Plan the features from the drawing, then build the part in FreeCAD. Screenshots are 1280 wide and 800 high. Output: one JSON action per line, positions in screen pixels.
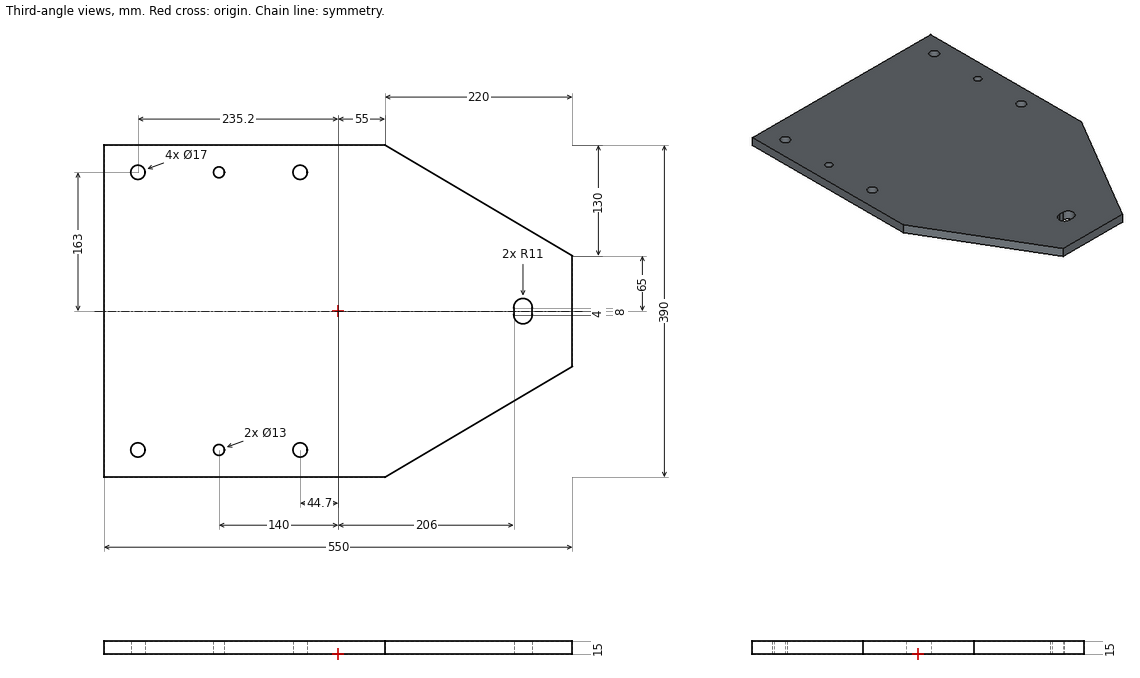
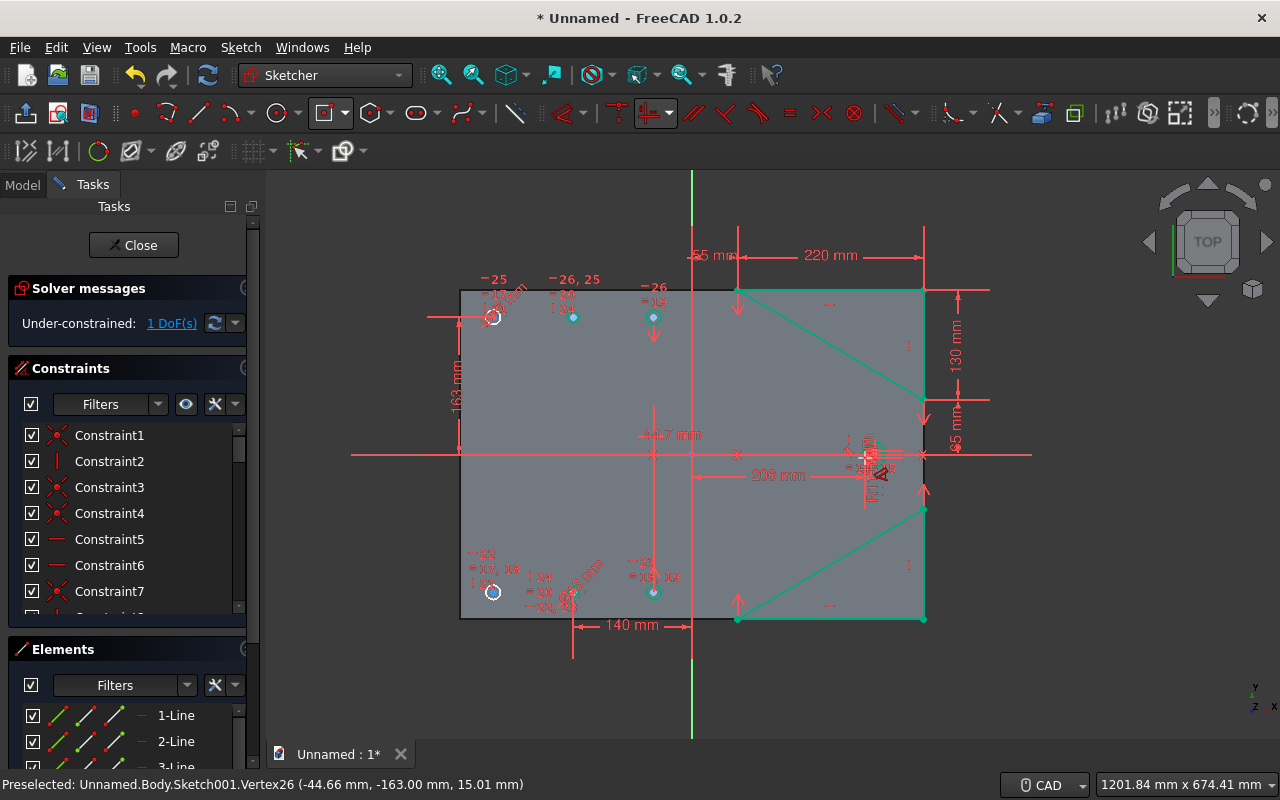
{"action": "left_click", "coordinate": [493, 317]}
{"action": "left_click", "coordinate": [592, 283]}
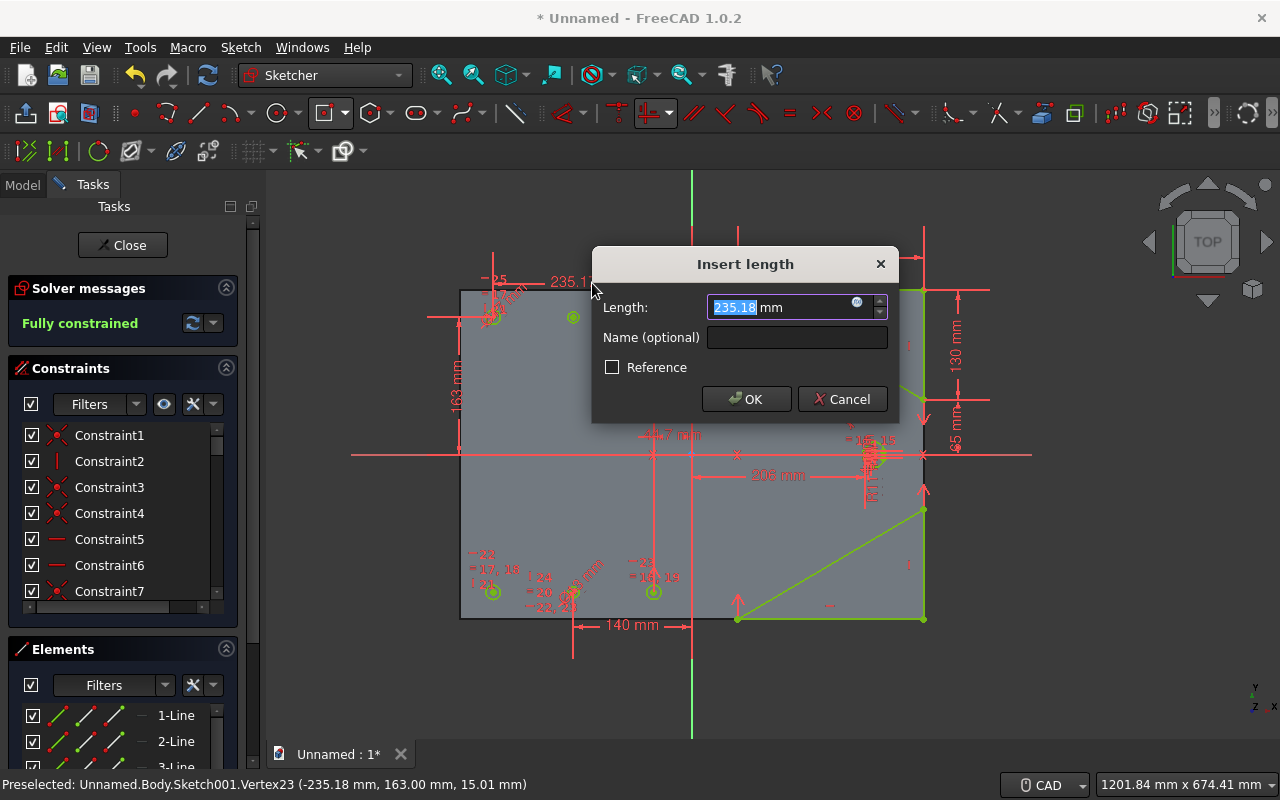
{"action": "type", "text": "235.2"}
{"action": "key", "text": "Return"}
{"action": "key", "text": "Escape"}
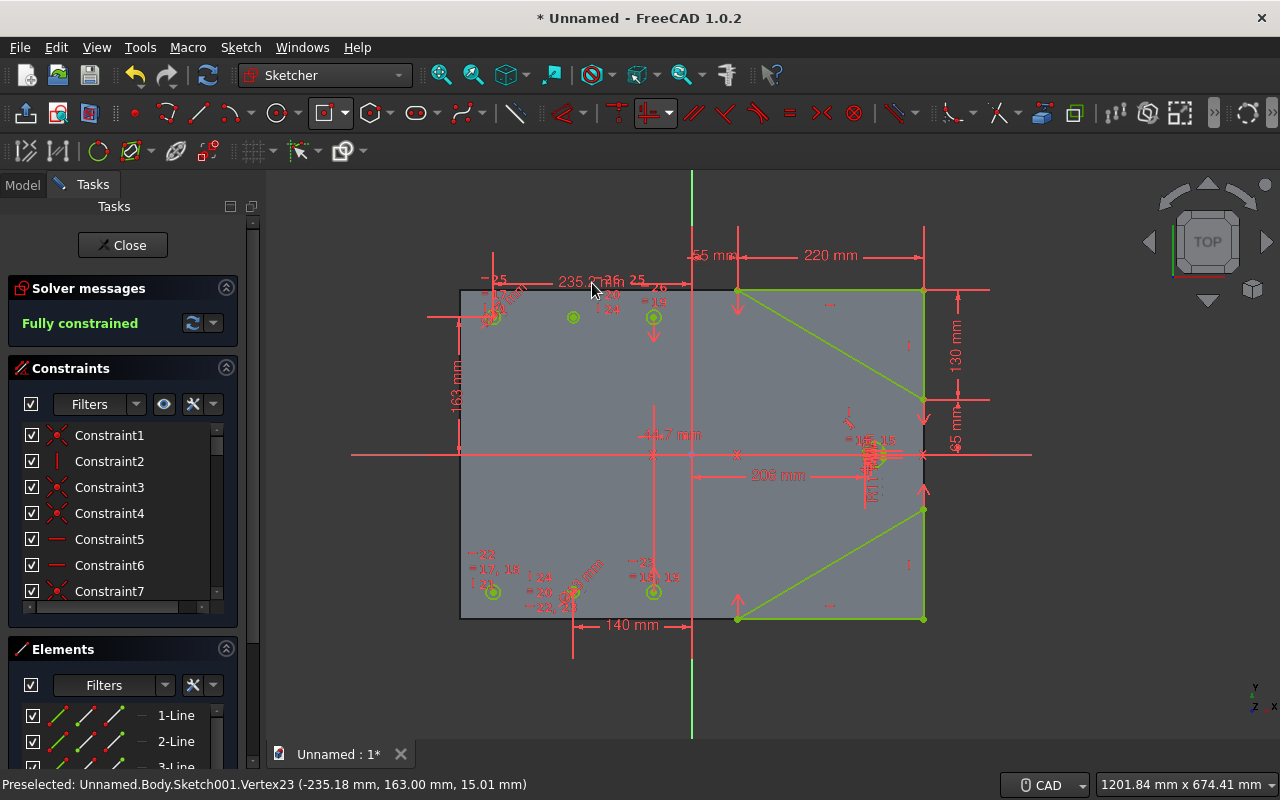
{"action": "left_click", "coordinate": [123, 245]}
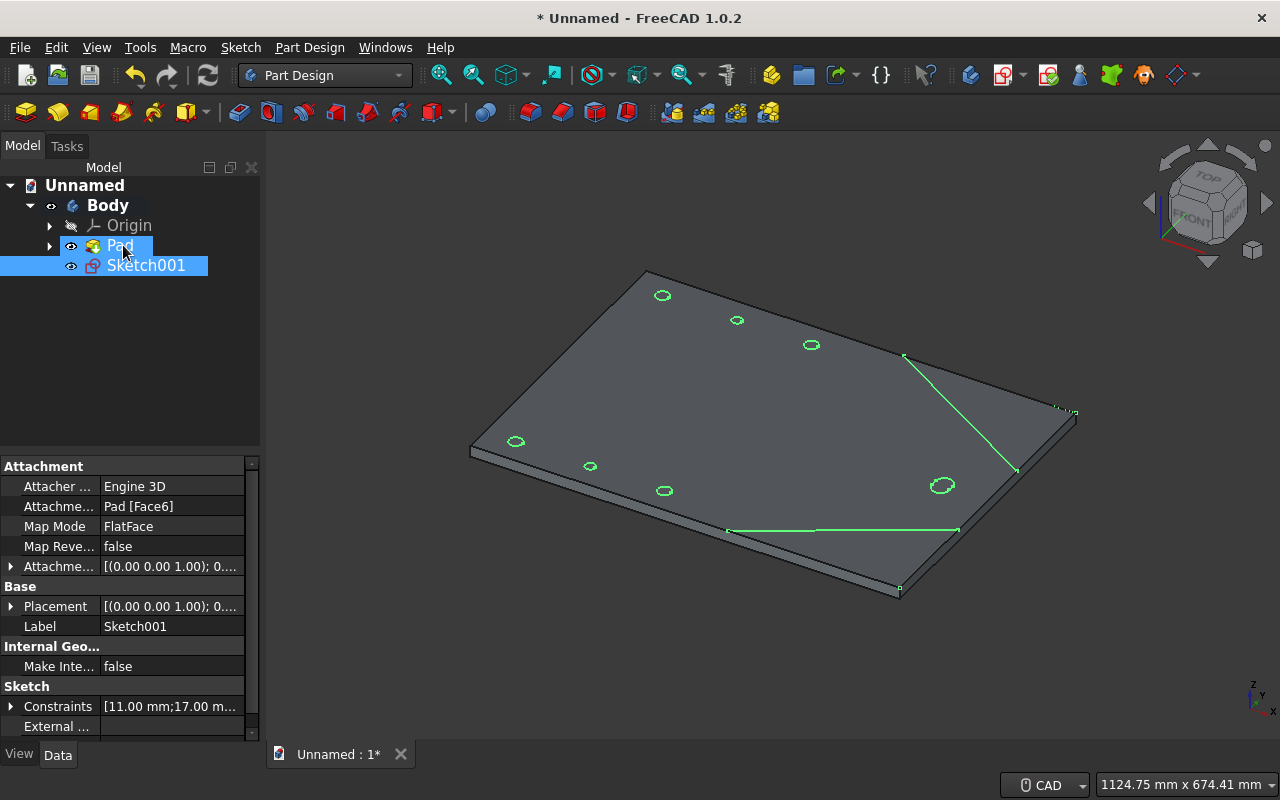
{"action": "left_click", "coordinate": [240, 112]}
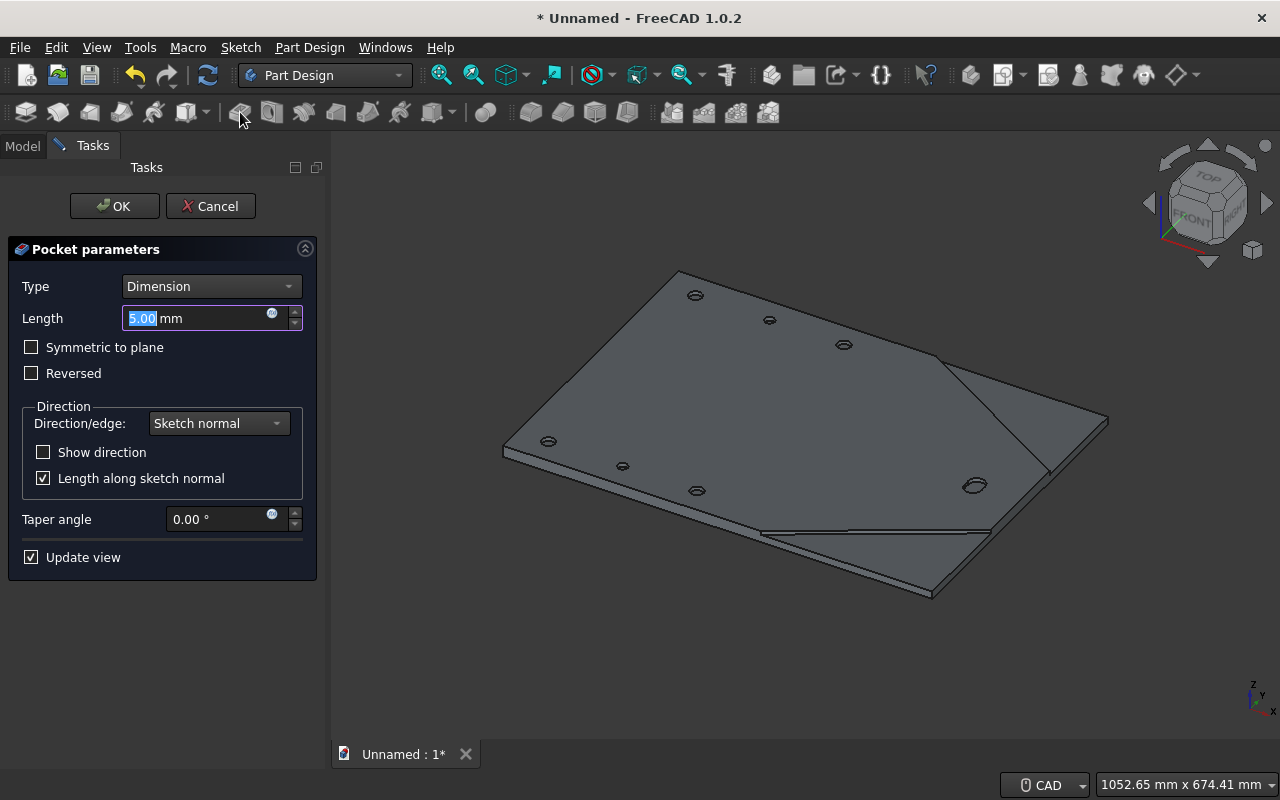
{"action": "type", "text": "15"}
{"action": "key", "text": "Tab"}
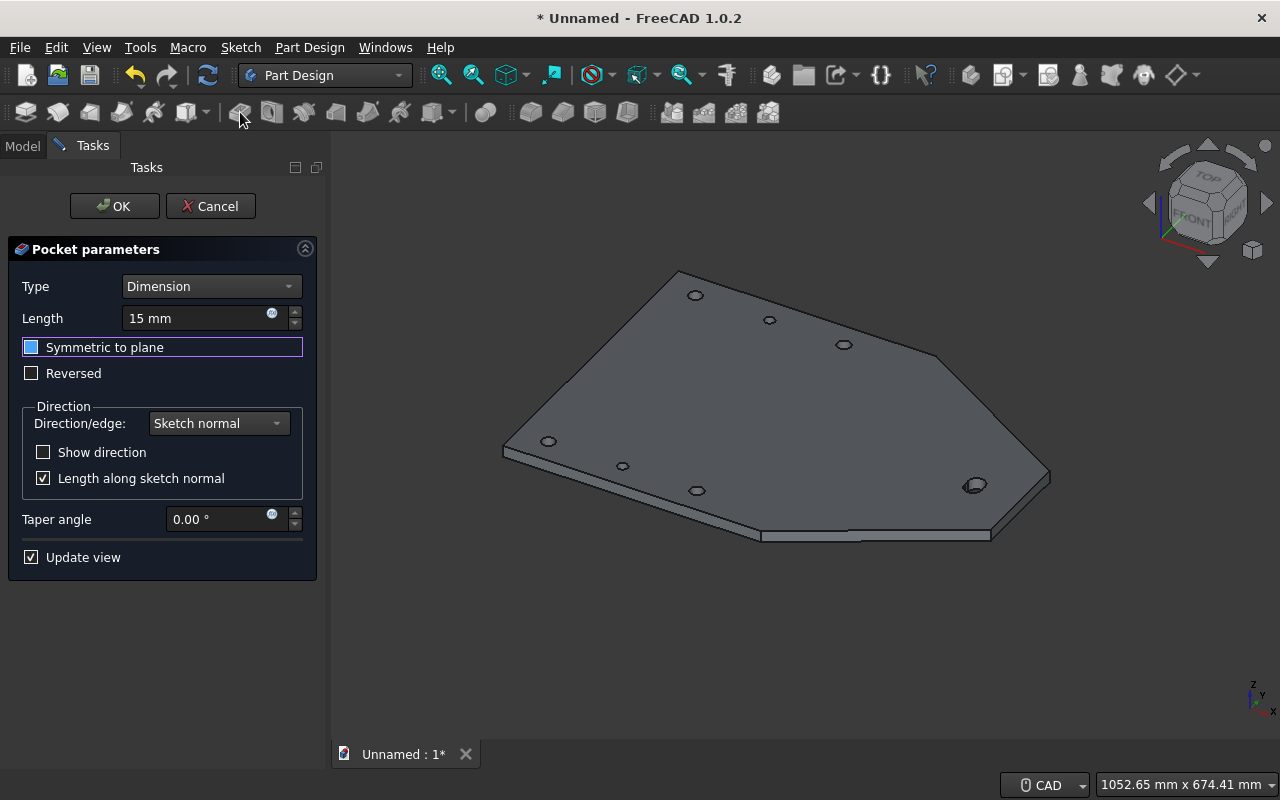
{"action": "left_click", "coordinate": [115, 206]}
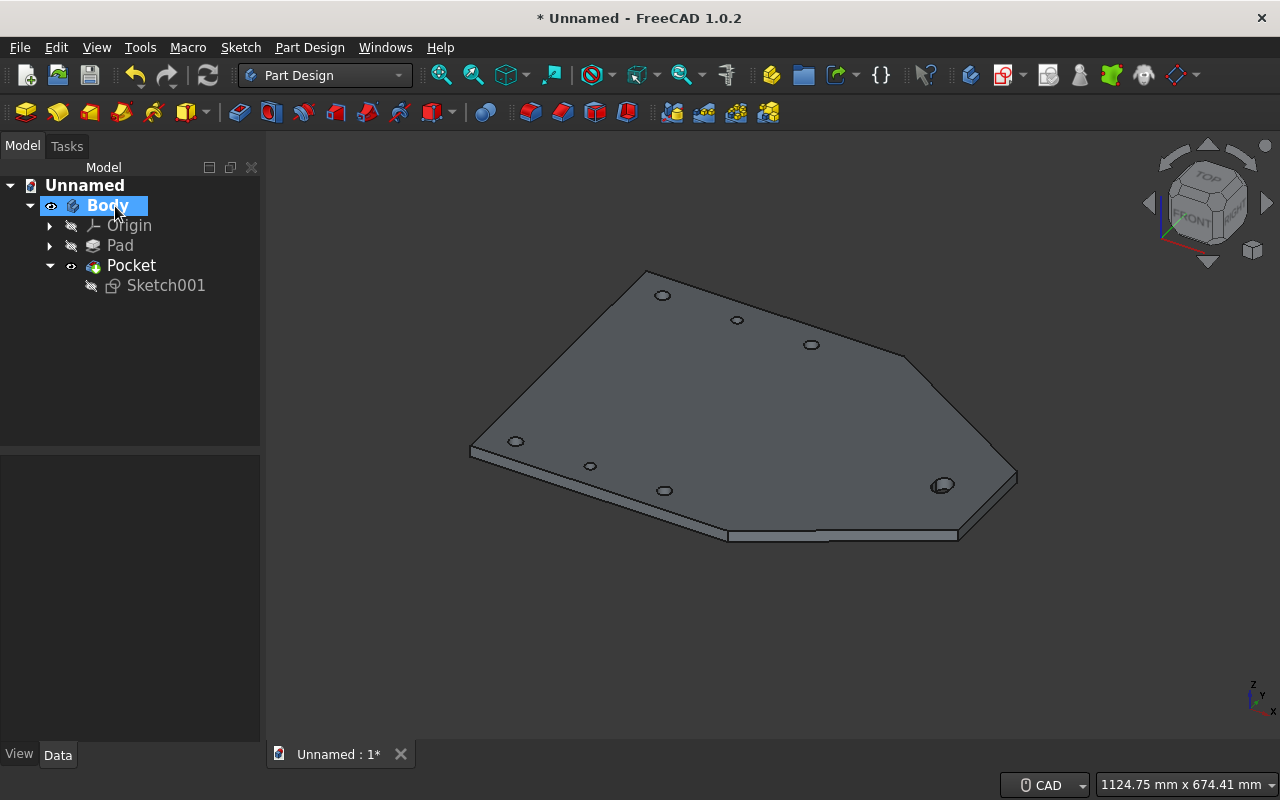
{"action": "key", "text": "0"}